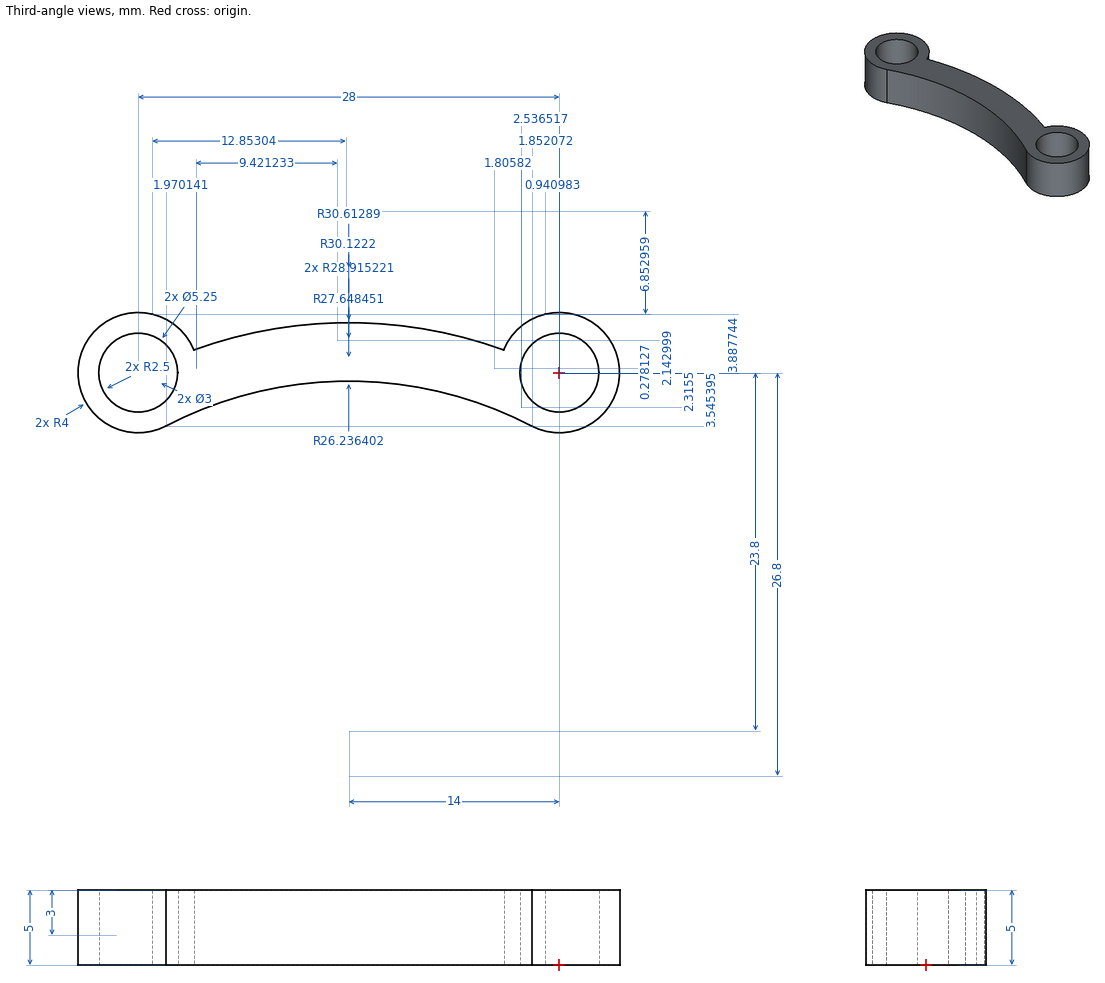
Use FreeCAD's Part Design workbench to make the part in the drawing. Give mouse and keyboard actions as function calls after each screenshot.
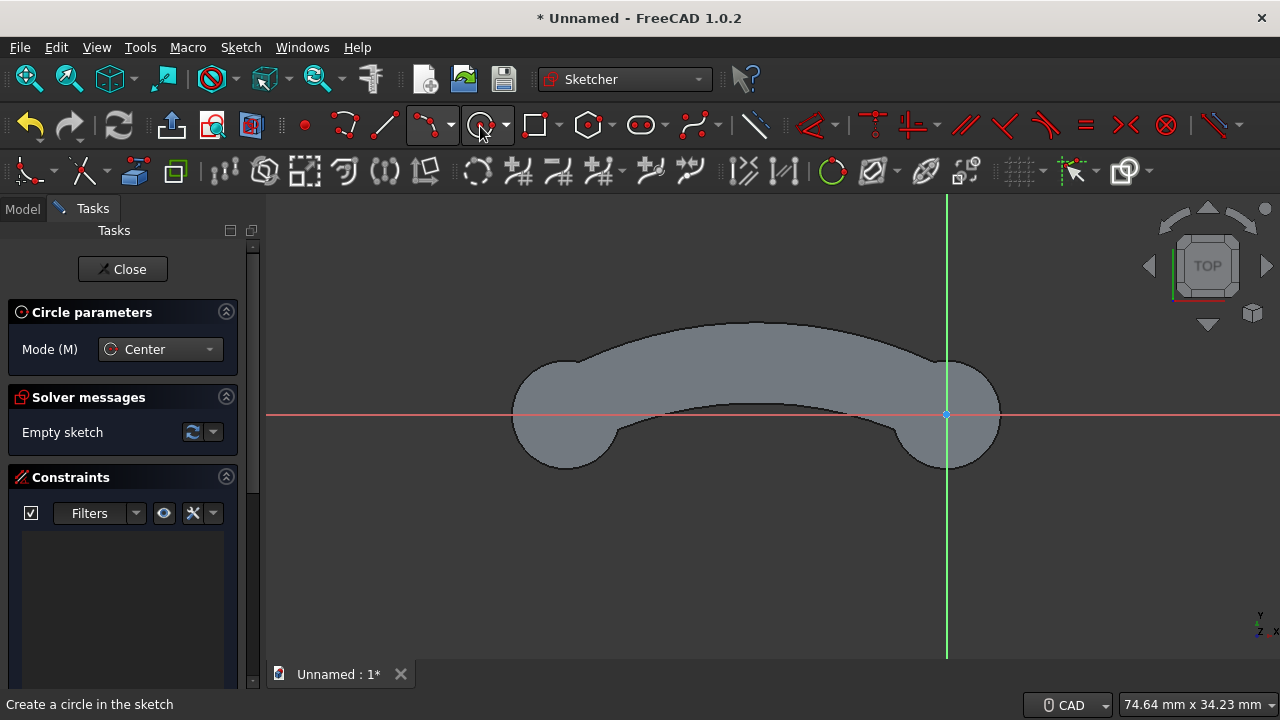
click(566, 415)
click(591, 390)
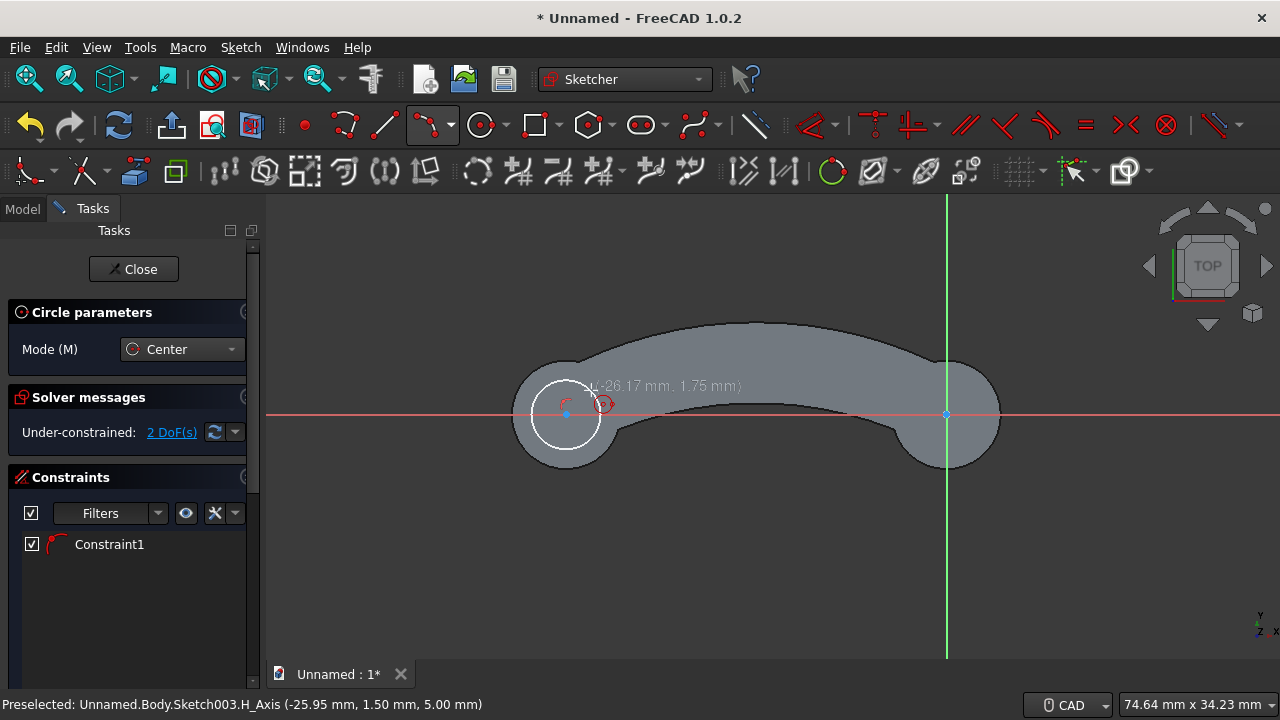
click(947, 415)
click(972, 390)
key(Escape)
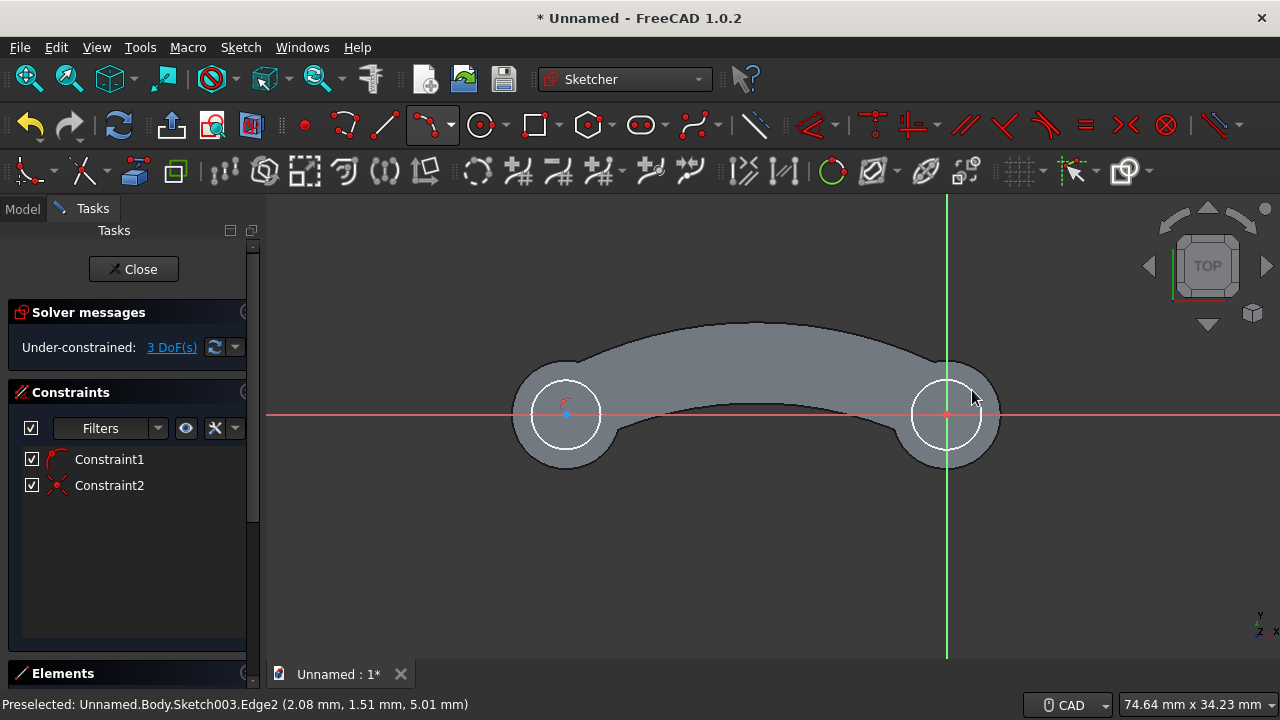
click(590, 390)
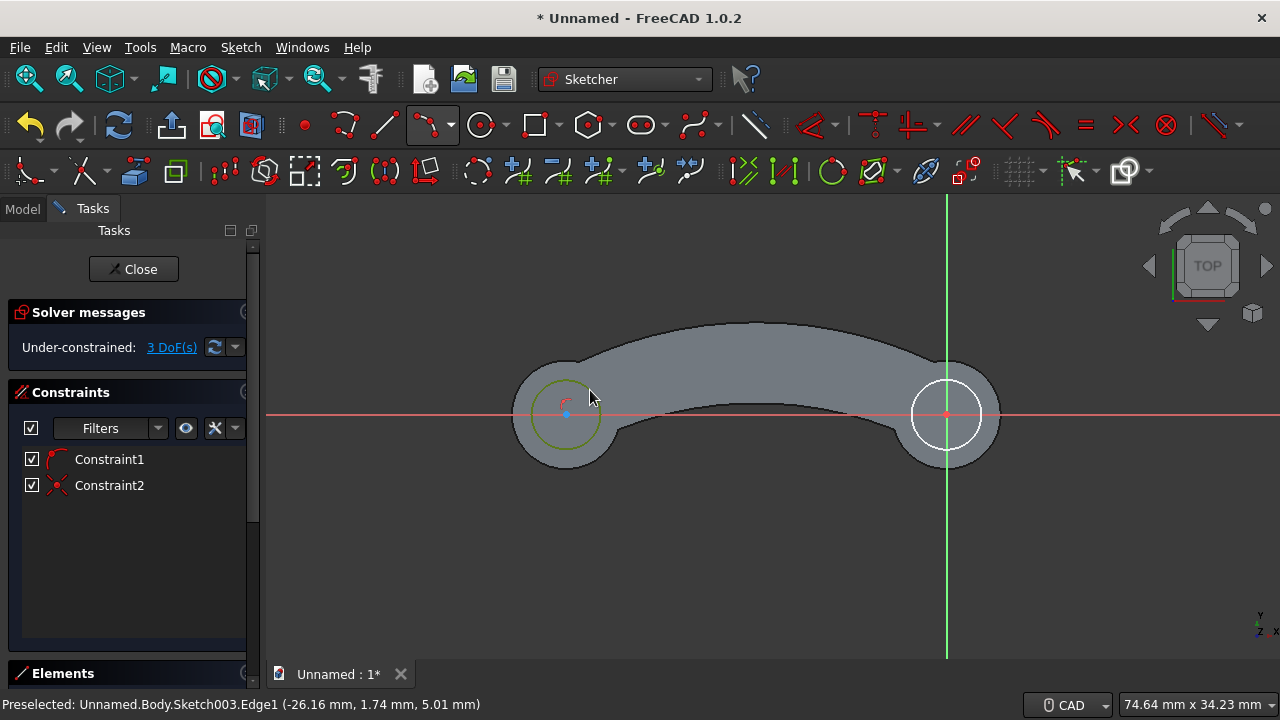
click(971, 390)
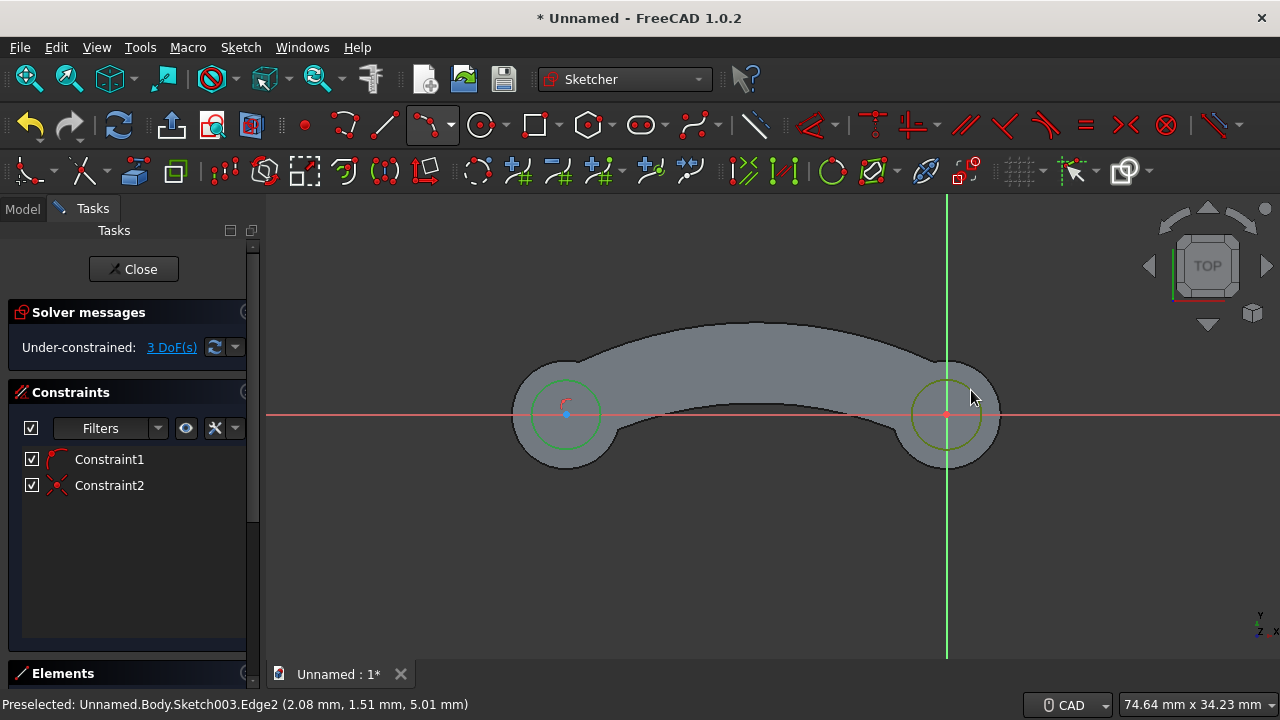
click(1086, 126)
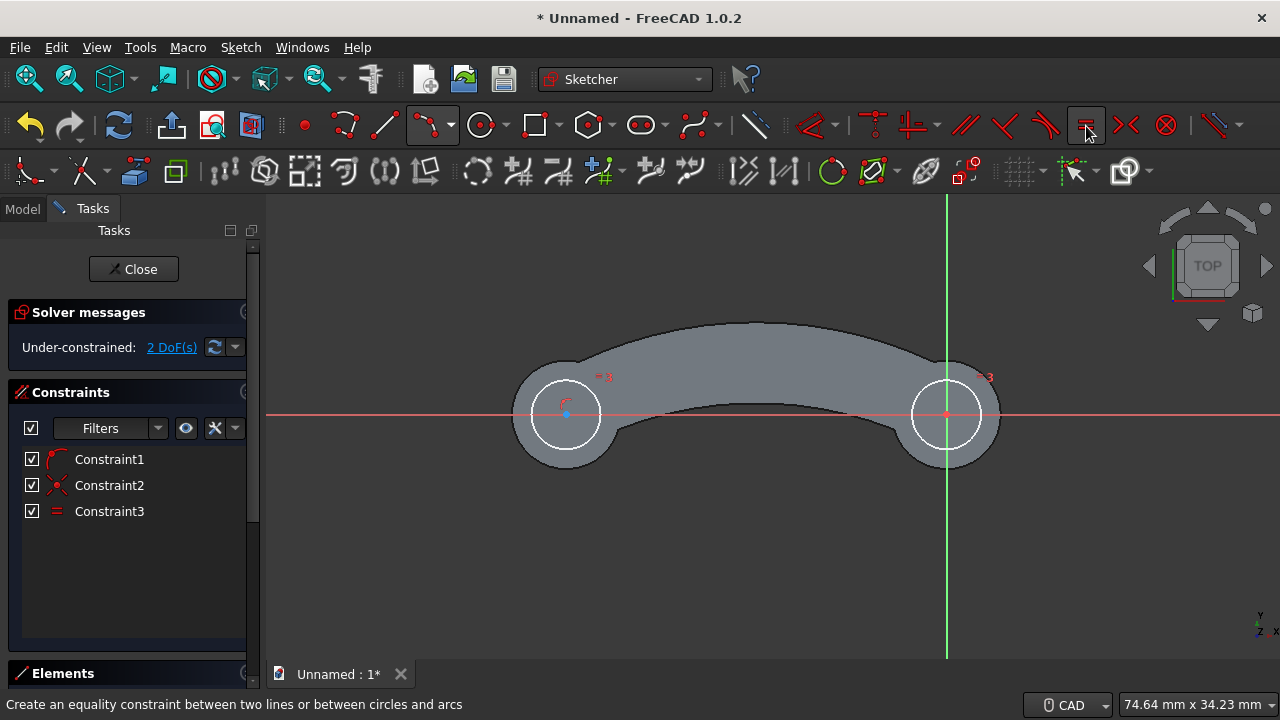
click(810, 126)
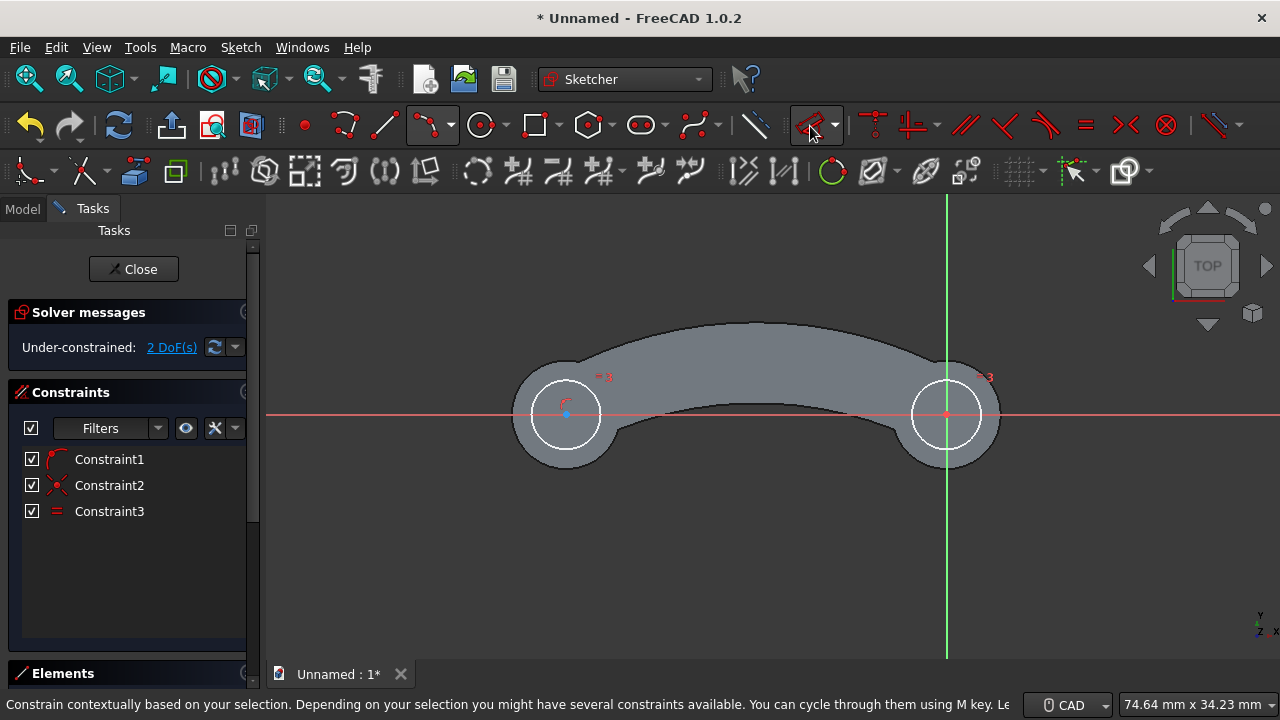
click(590, 390)
click(612, 367)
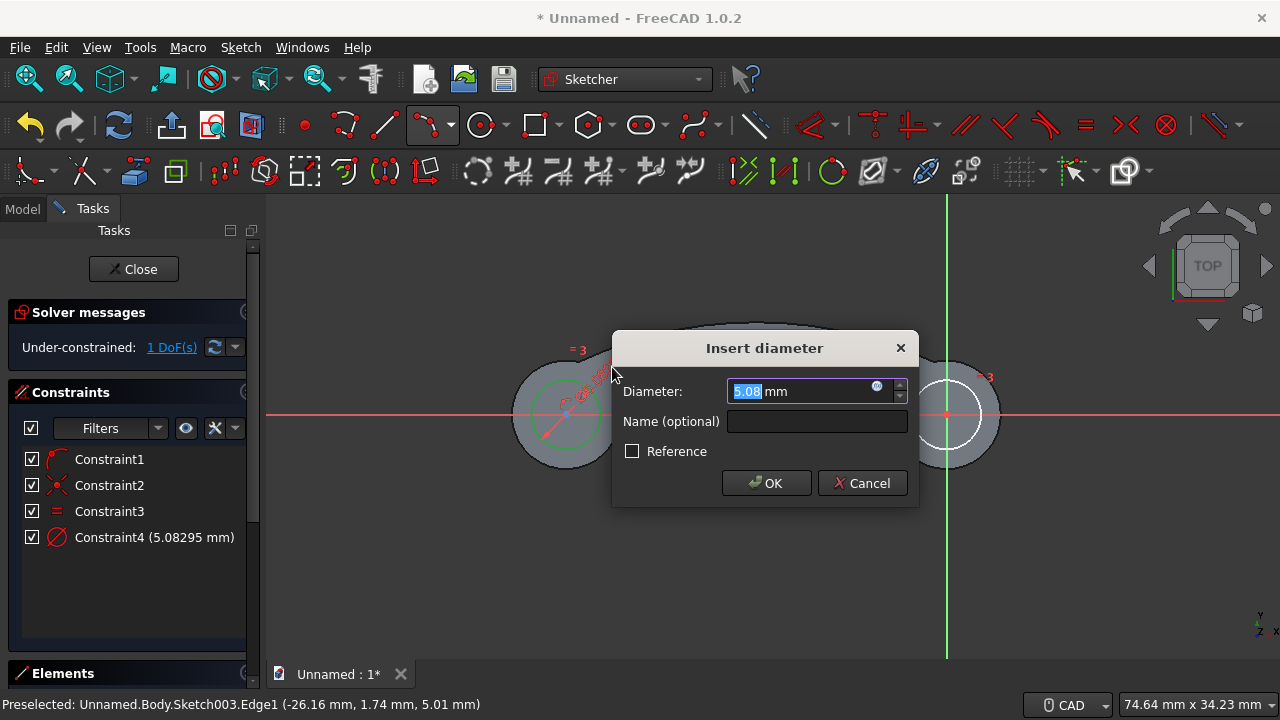
text(5.25)
key(Return)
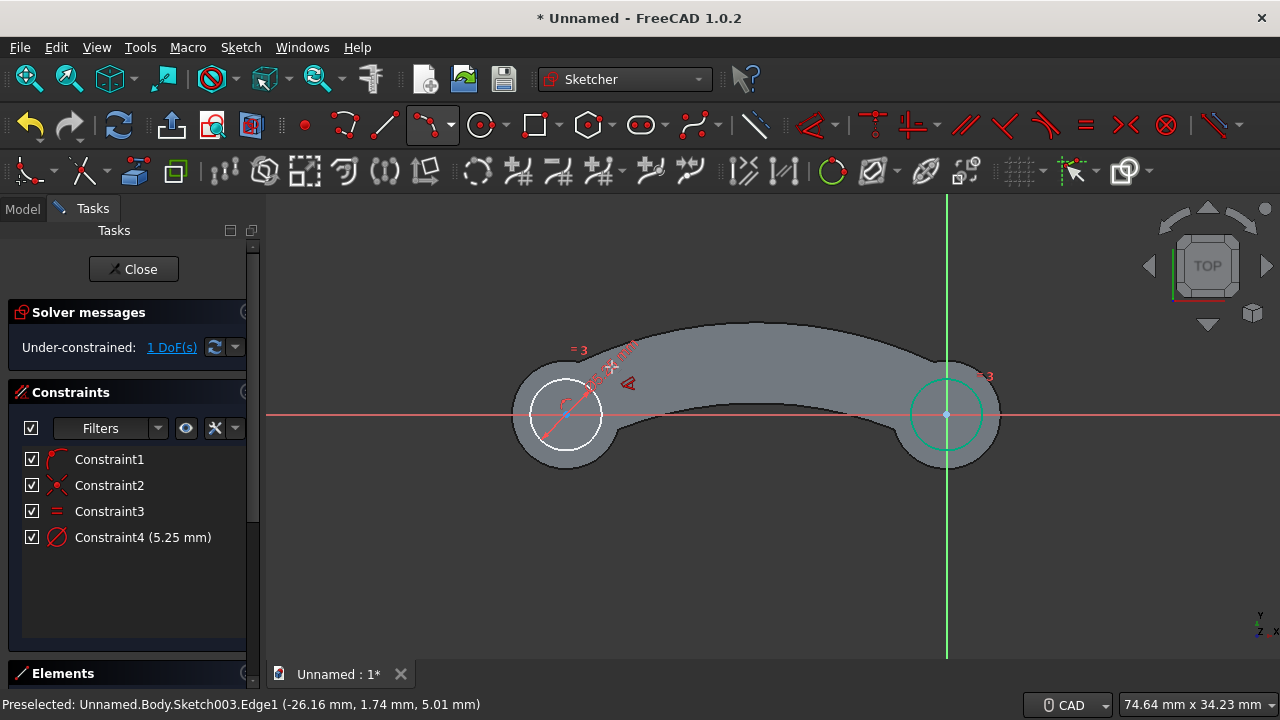
click(566, 415)
click(756, 449)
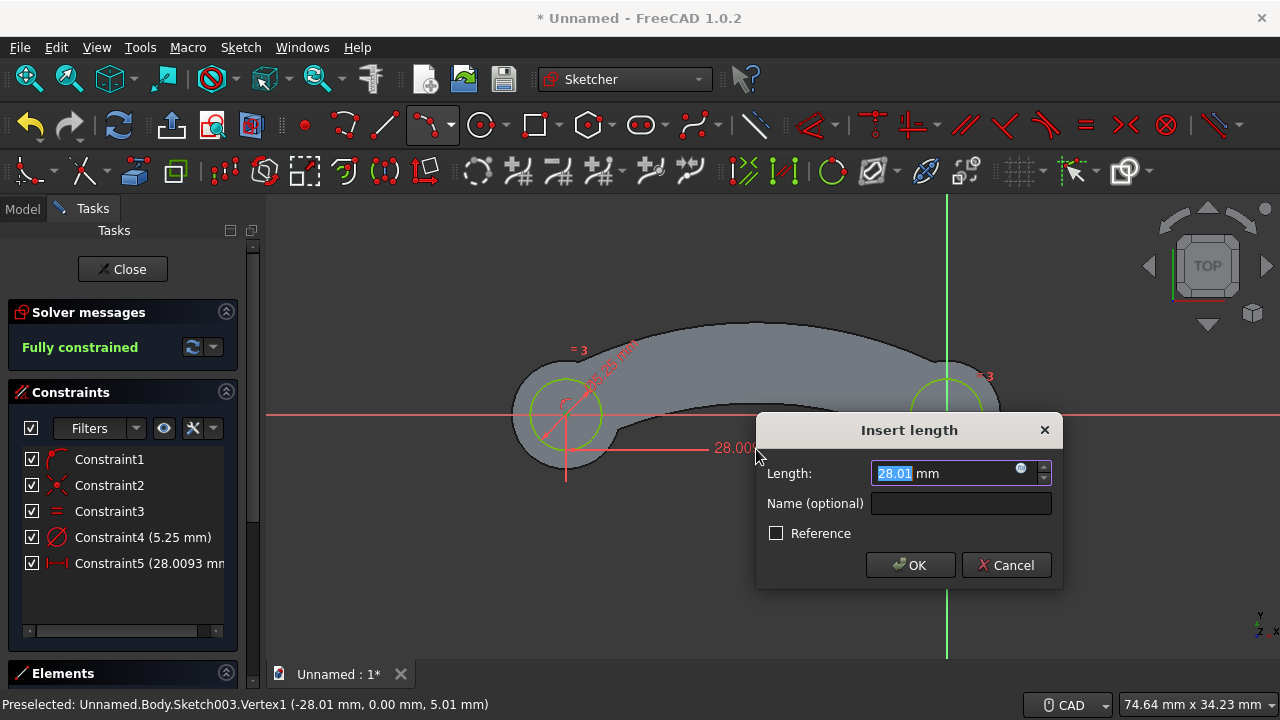
text(28)
key(Return)
key(Escape)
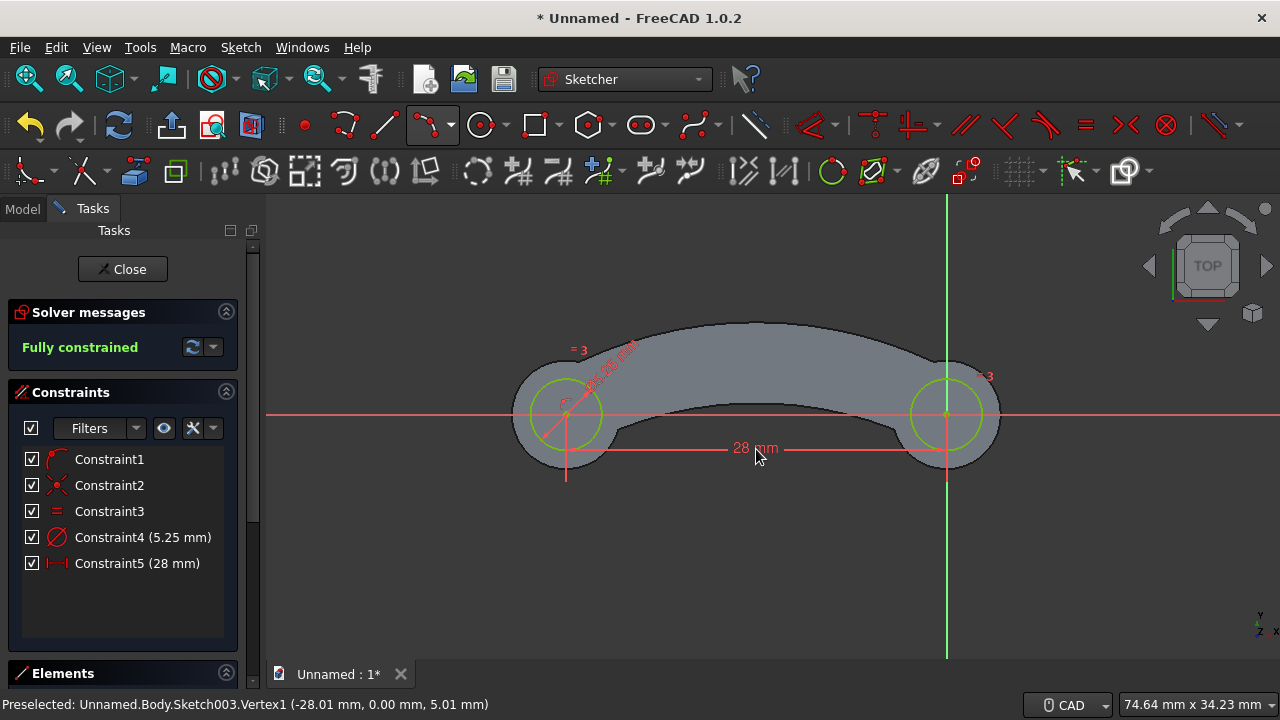
click(123, 269)